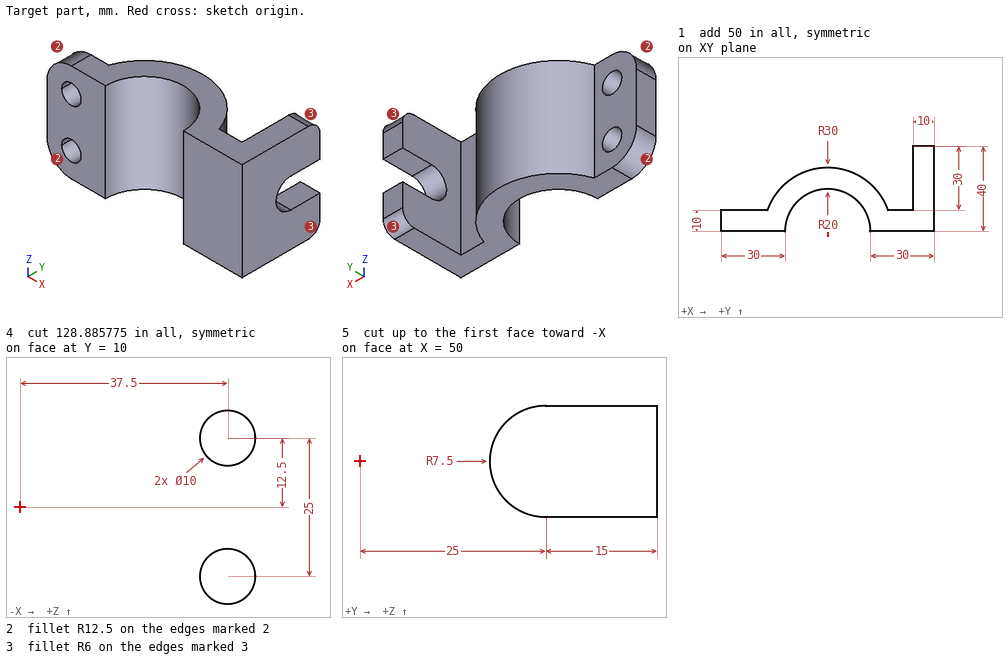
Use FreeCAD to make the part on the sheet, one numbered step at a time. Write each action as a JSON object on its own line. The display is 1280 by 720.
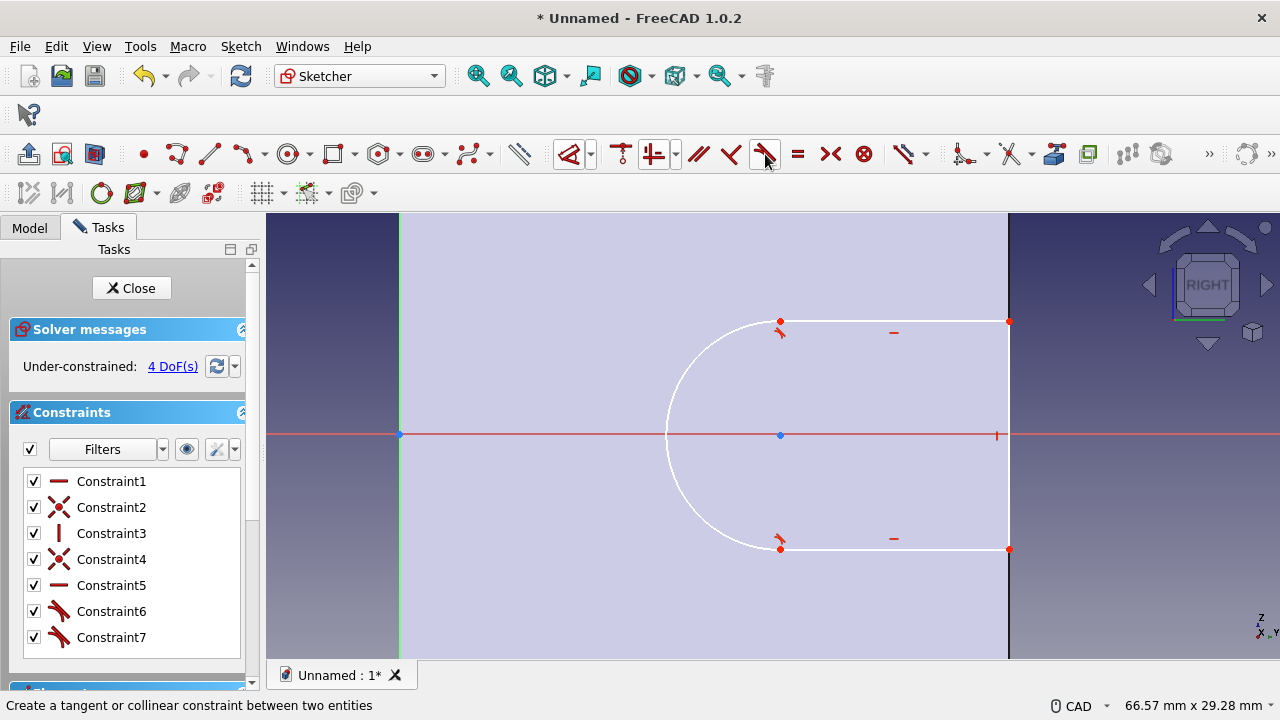
{"action": "left_click", "coordinate": [781, 436]}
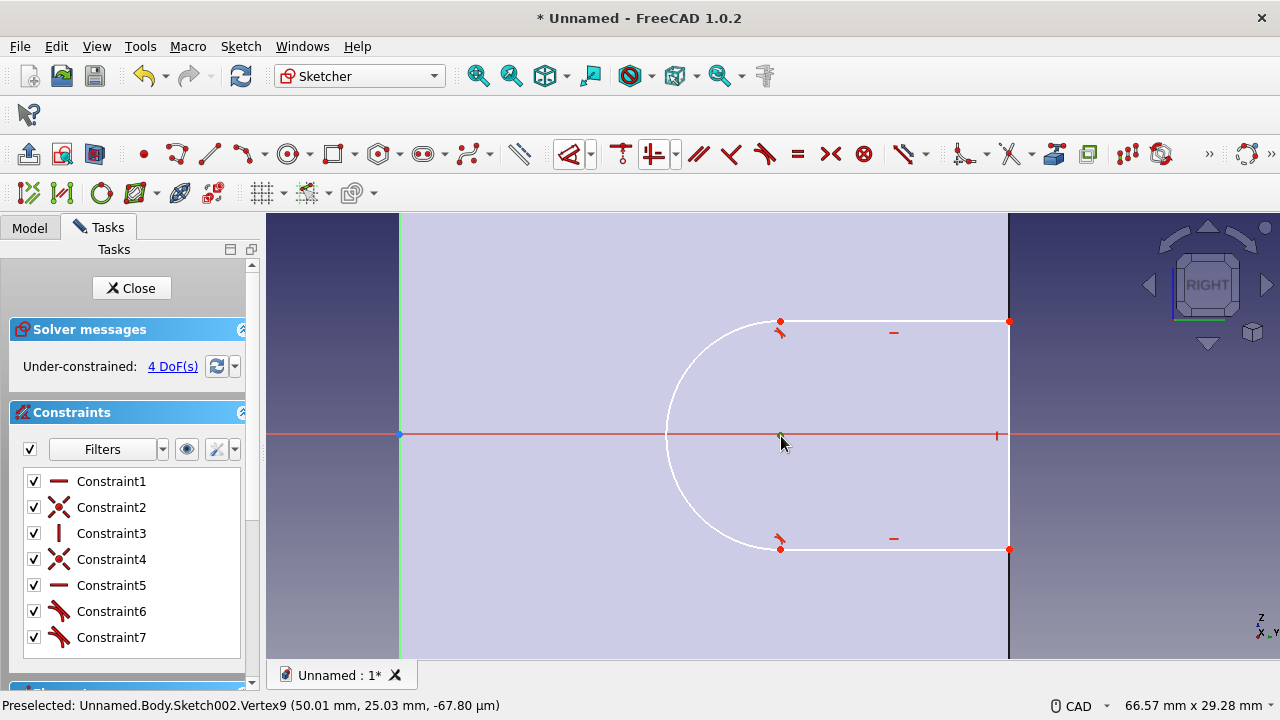
{"action": "left_click", "coordinate": [353, 434]}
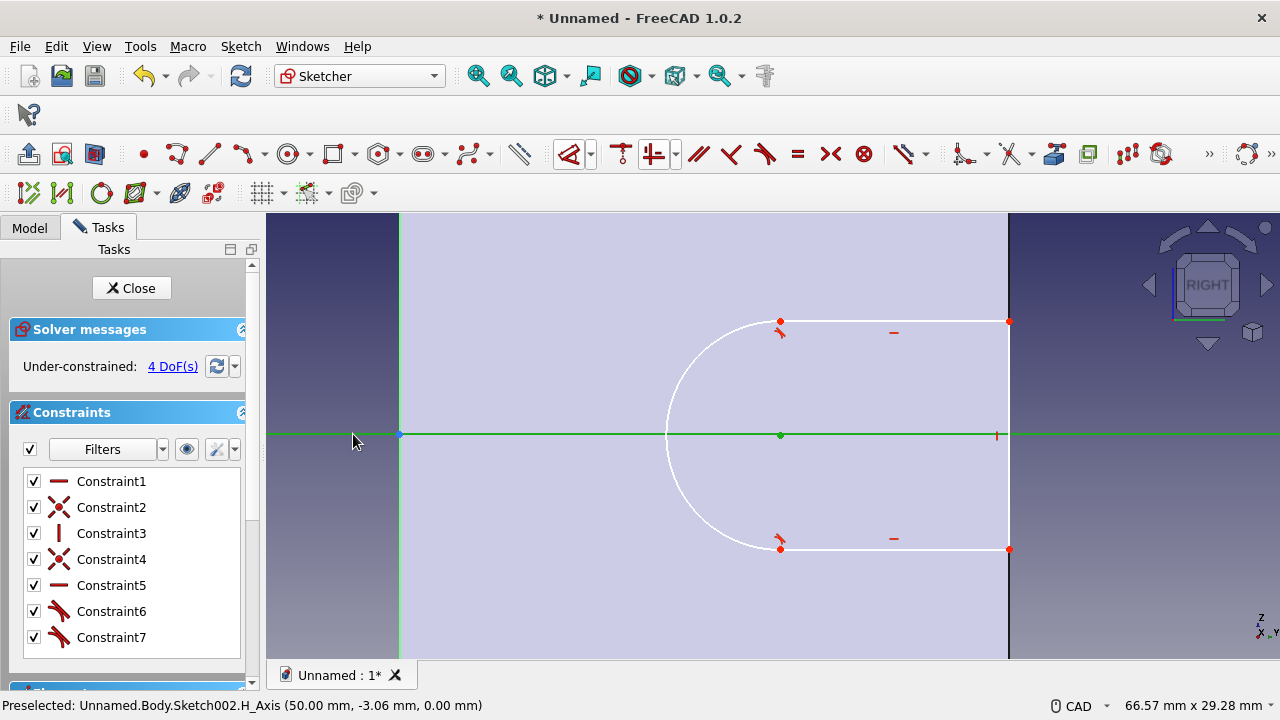
{"action": "left_click", "coordinate": [621, 154]}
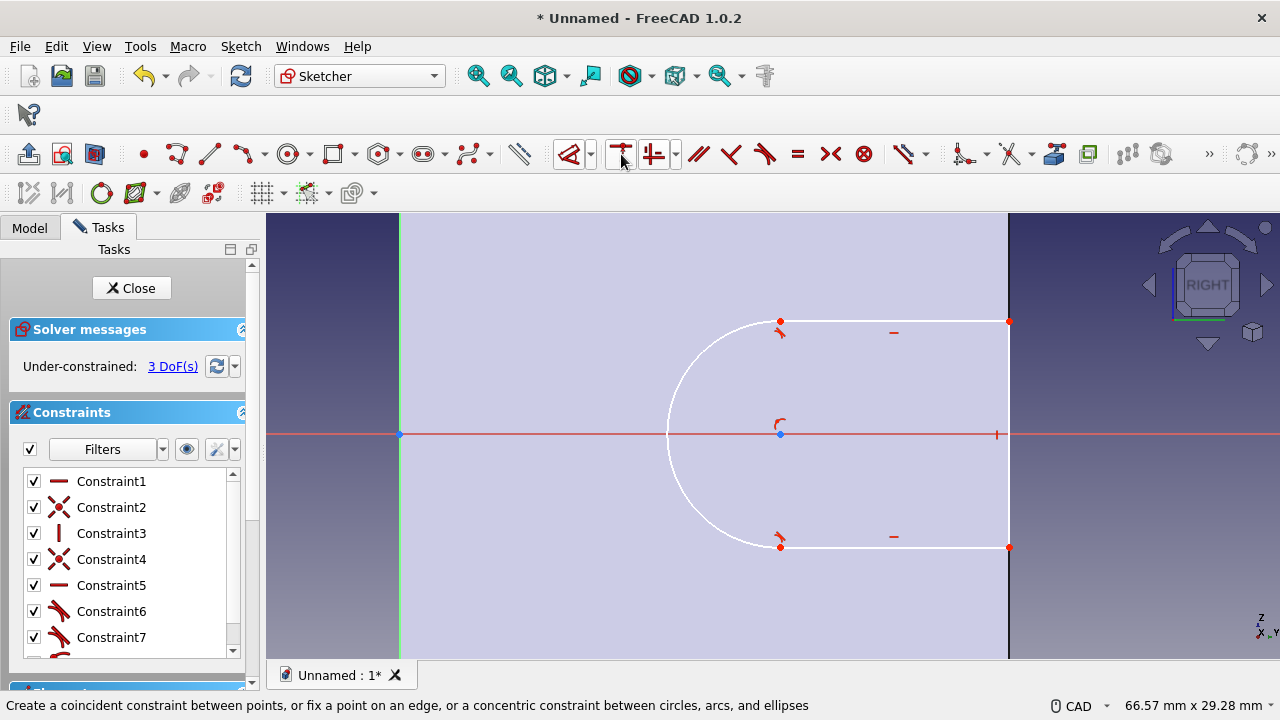
{"action": "left_click", "coordinate": [689, 368]}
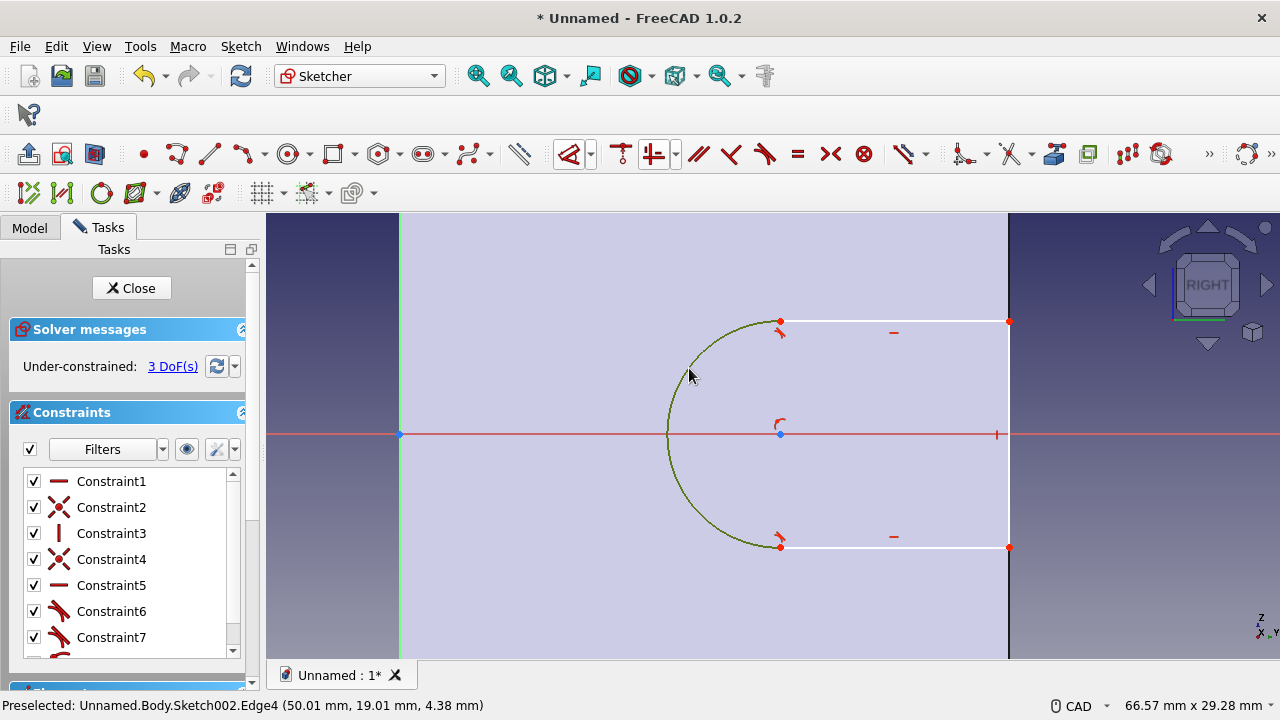
{"action": "left_click", "coordinate": [590, 154]}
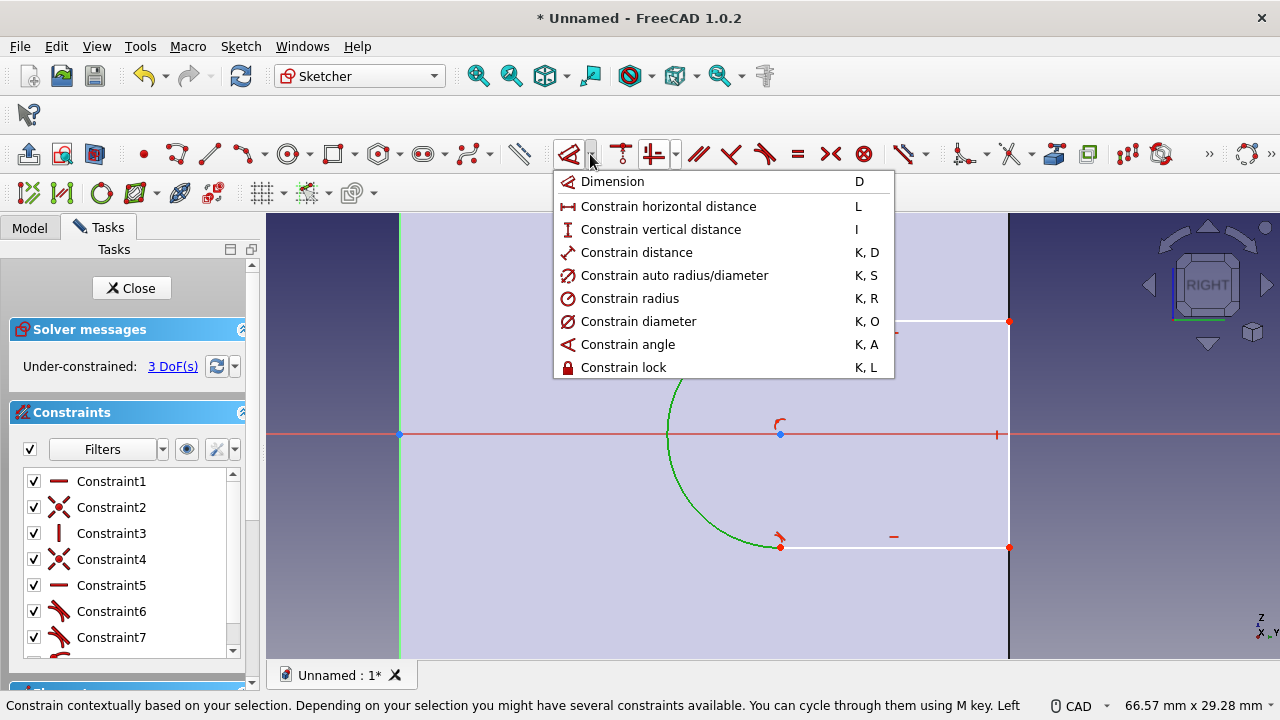
{"action": "left_click", "coordinate": [724, 298]}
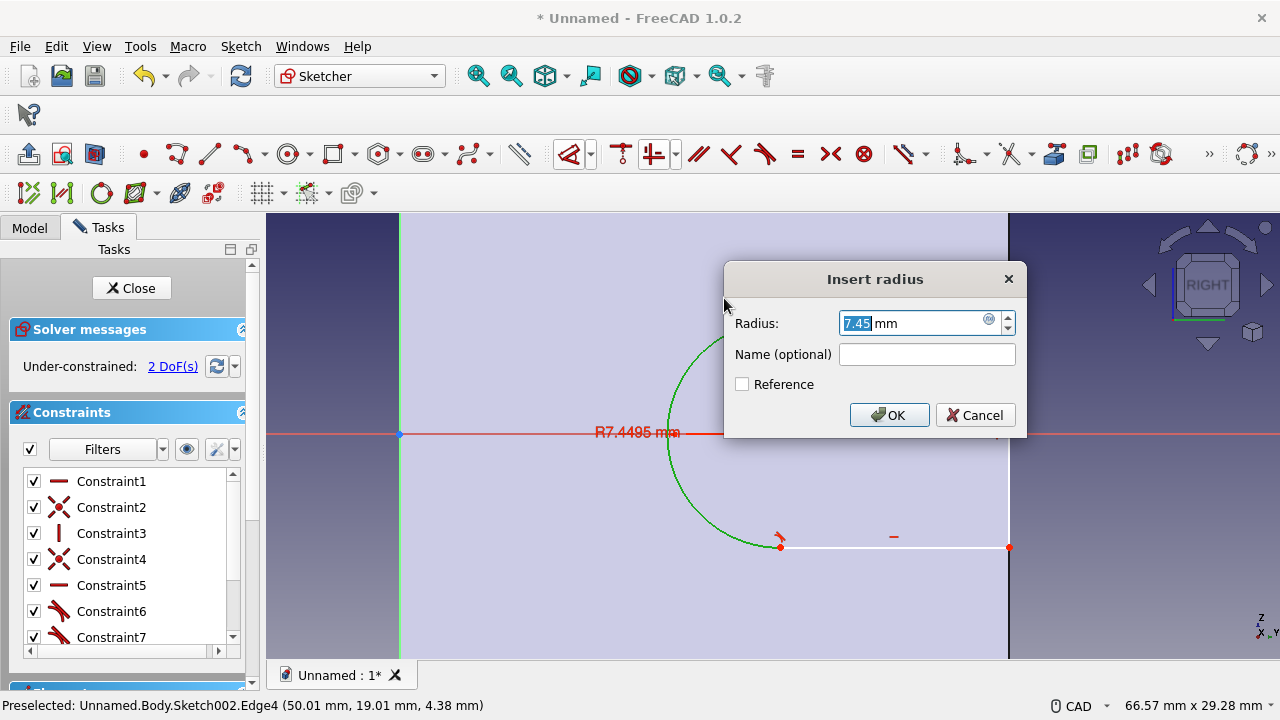
{"action": "type", "text": "7.5"}
{"action": "key", "text": "Return"}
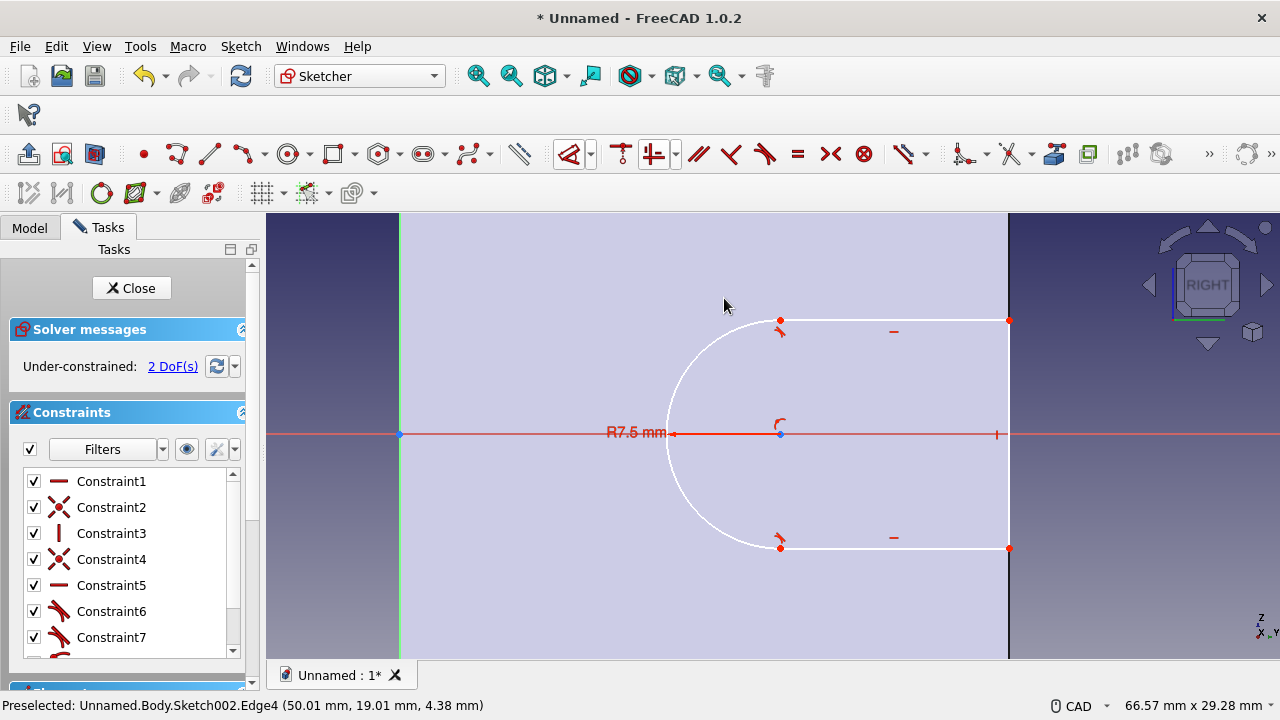
{"action": "left_click", "coordinate": [849, 549]}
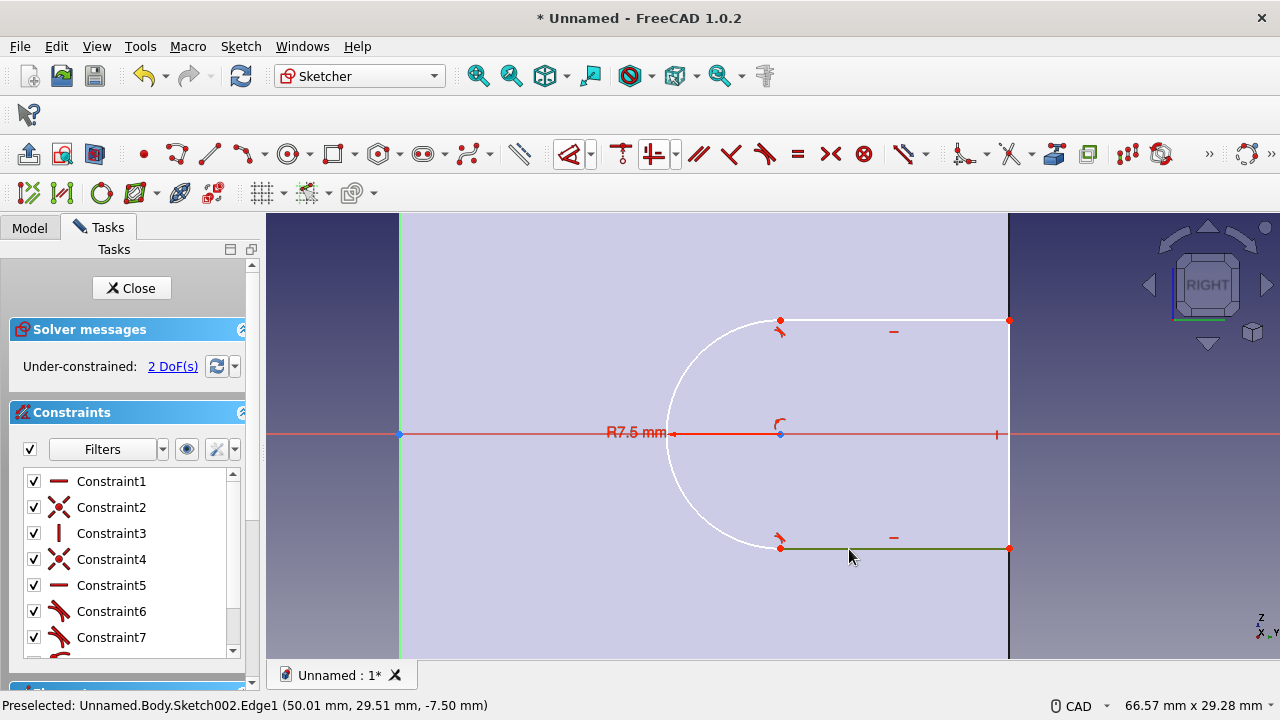
{"action": "key", "text": "l"}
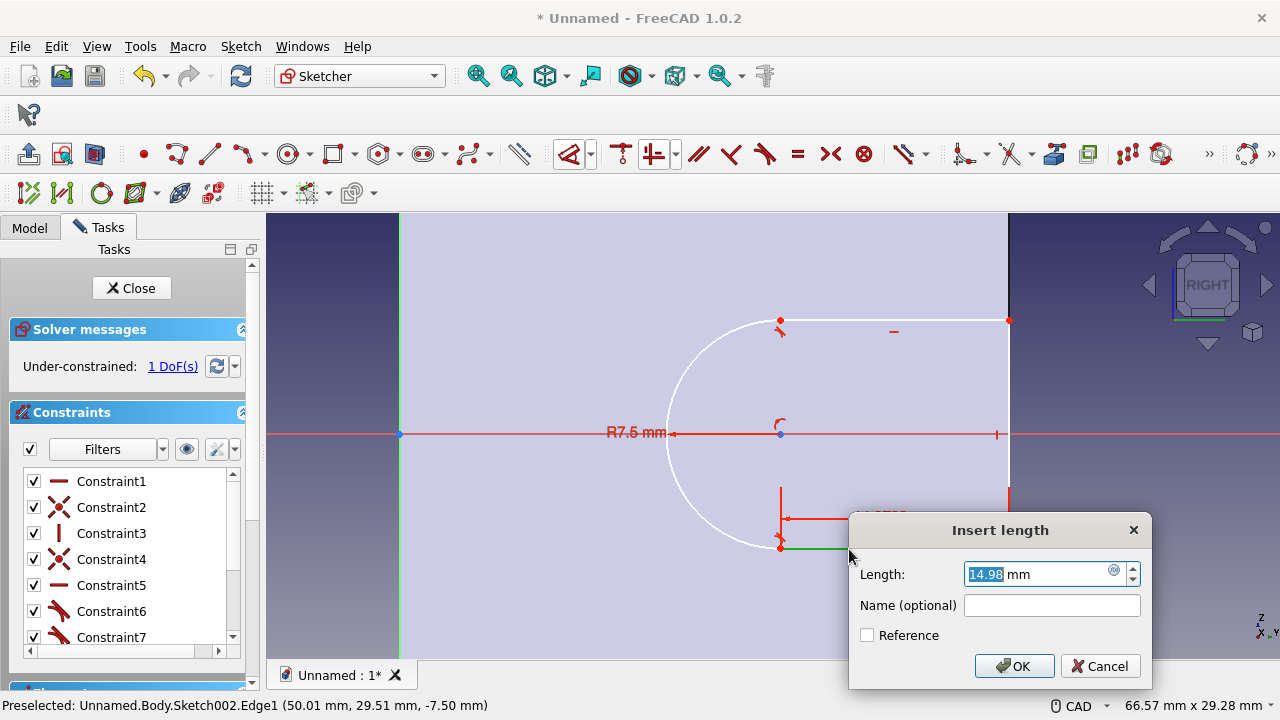
{"action": "type", "text": "15"}
{"action": "key", "text": "Return"}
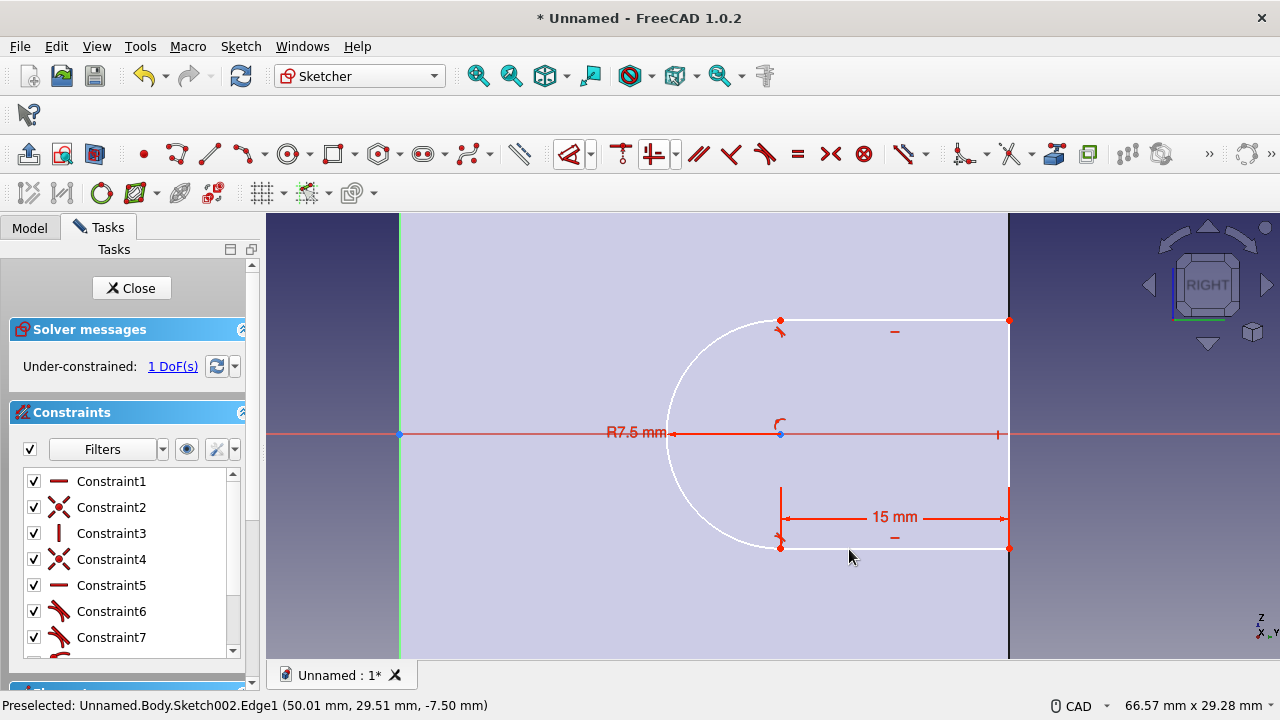
{"action": "left_click", "coordinate": [781, 549]}